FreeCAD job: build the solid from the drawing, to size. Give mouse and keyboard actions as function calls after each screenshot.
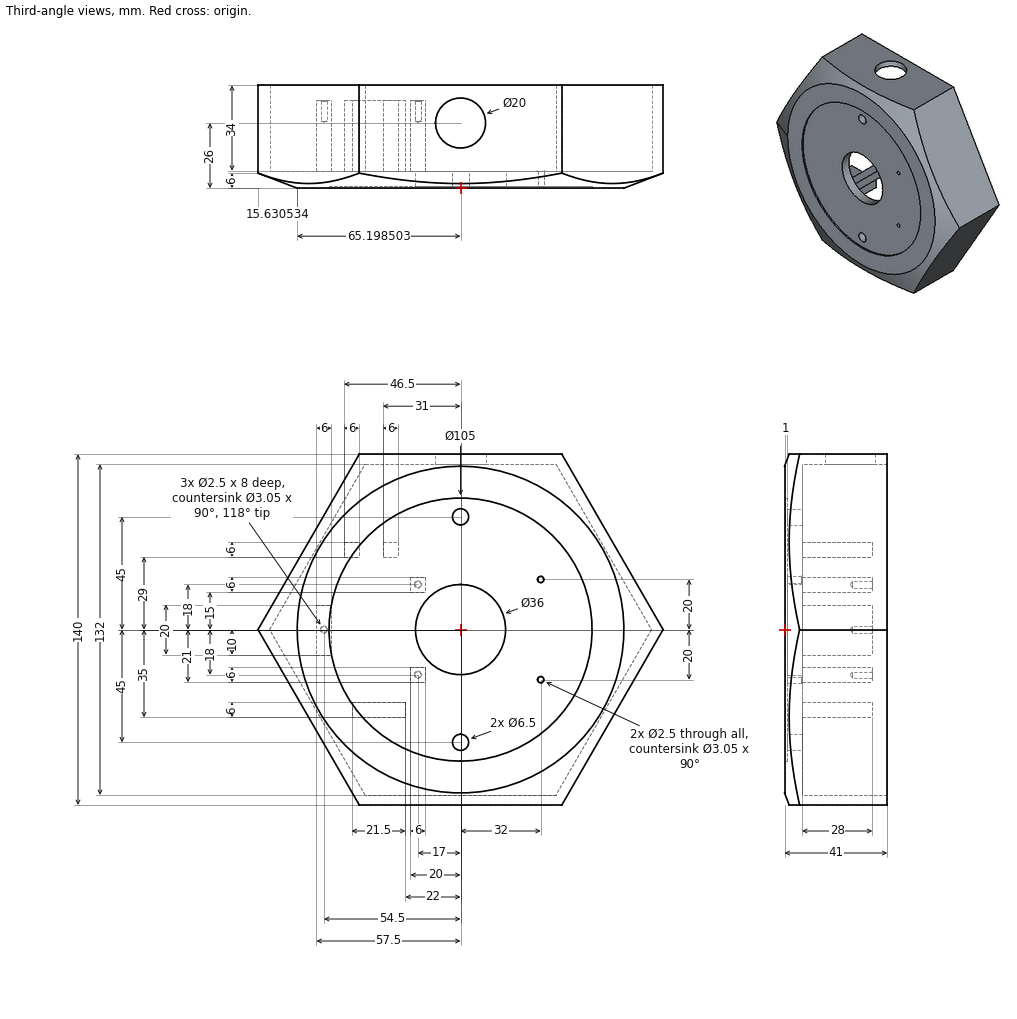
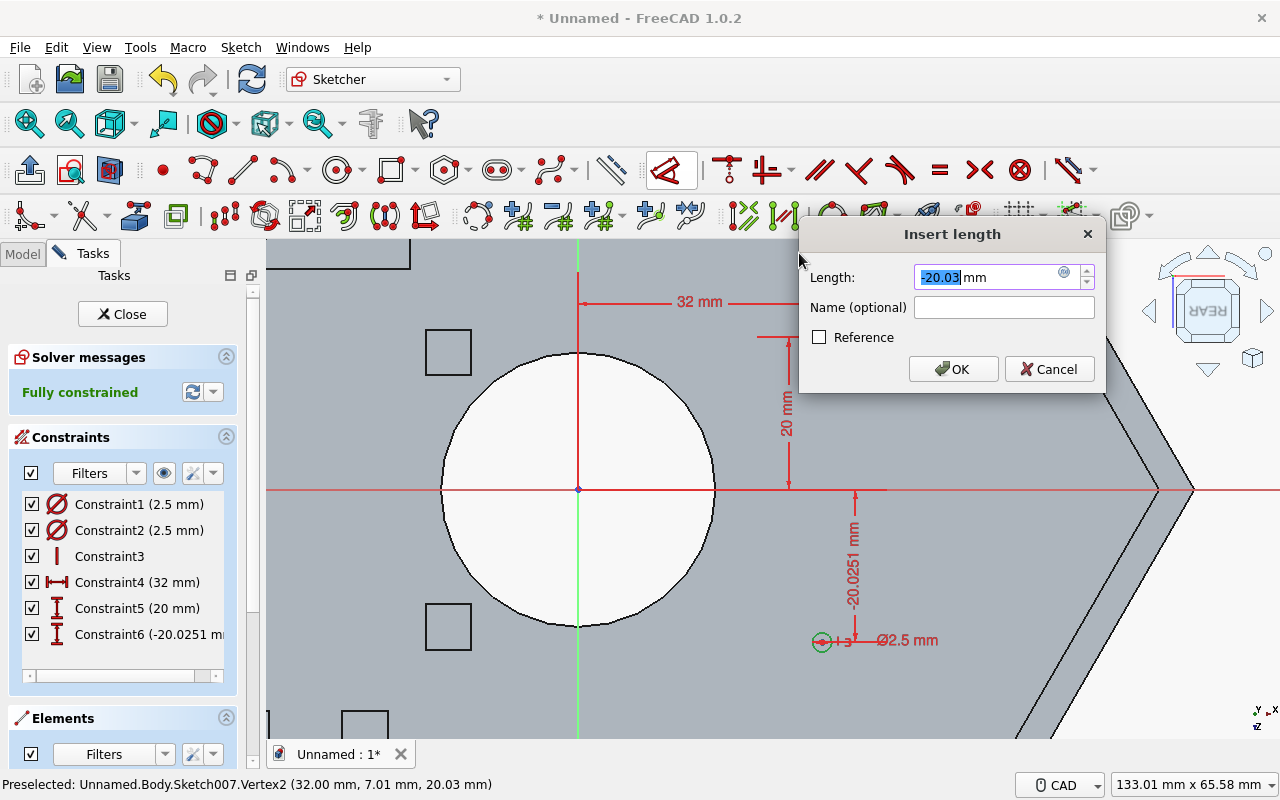
text(-20)
key(Return)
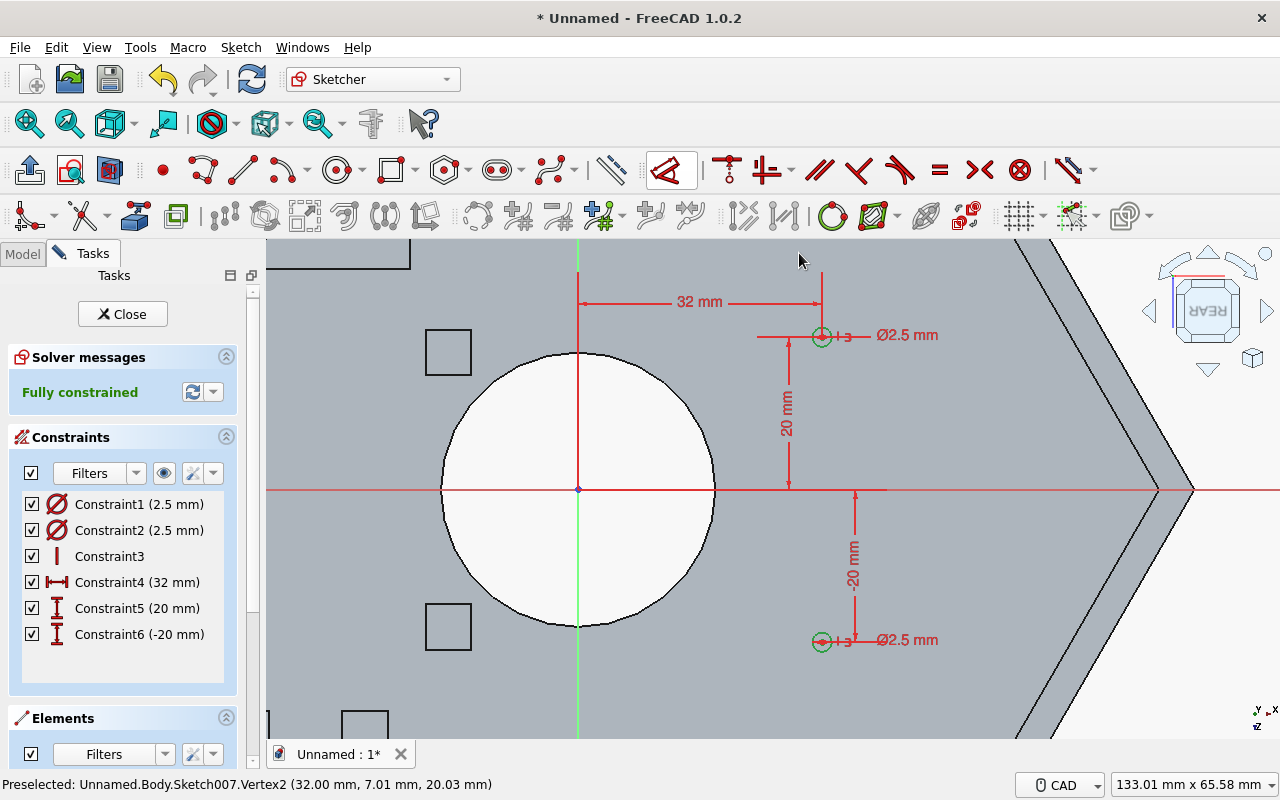
click(123, 314)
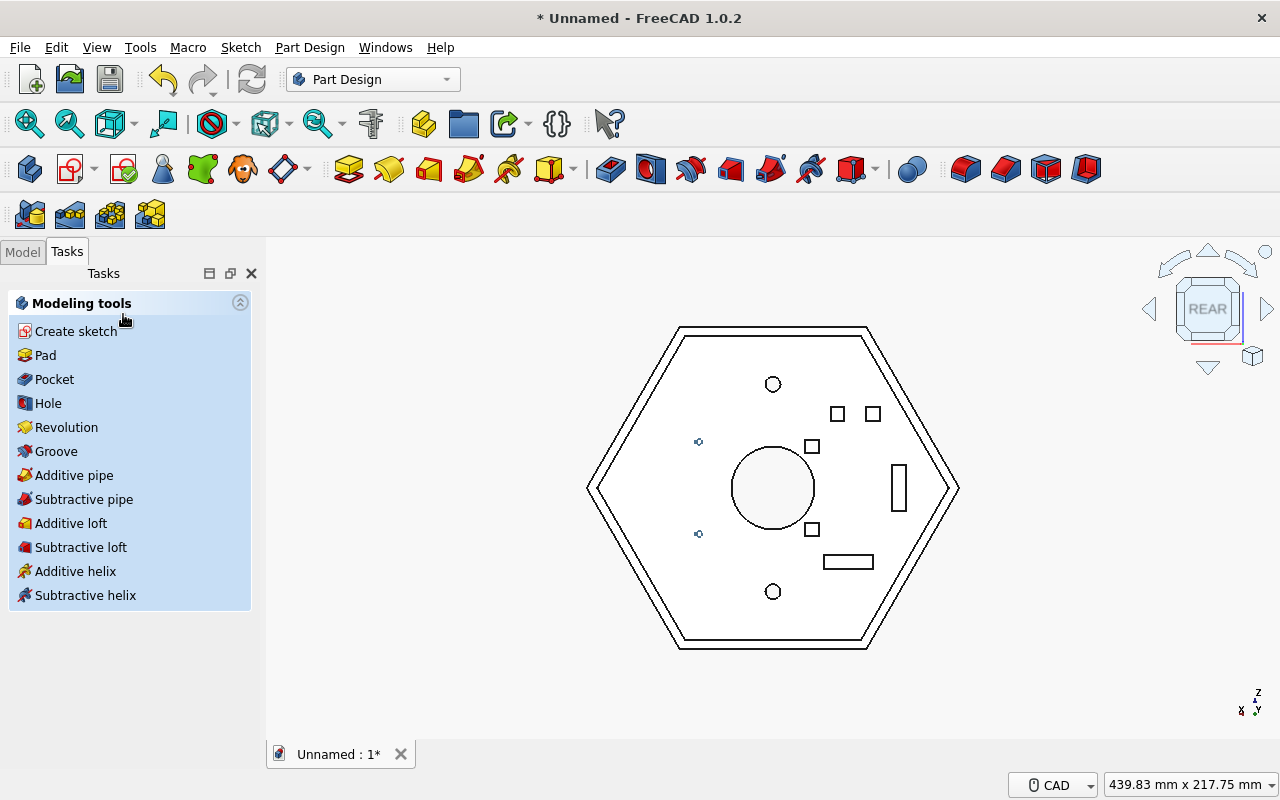
click(652, 170)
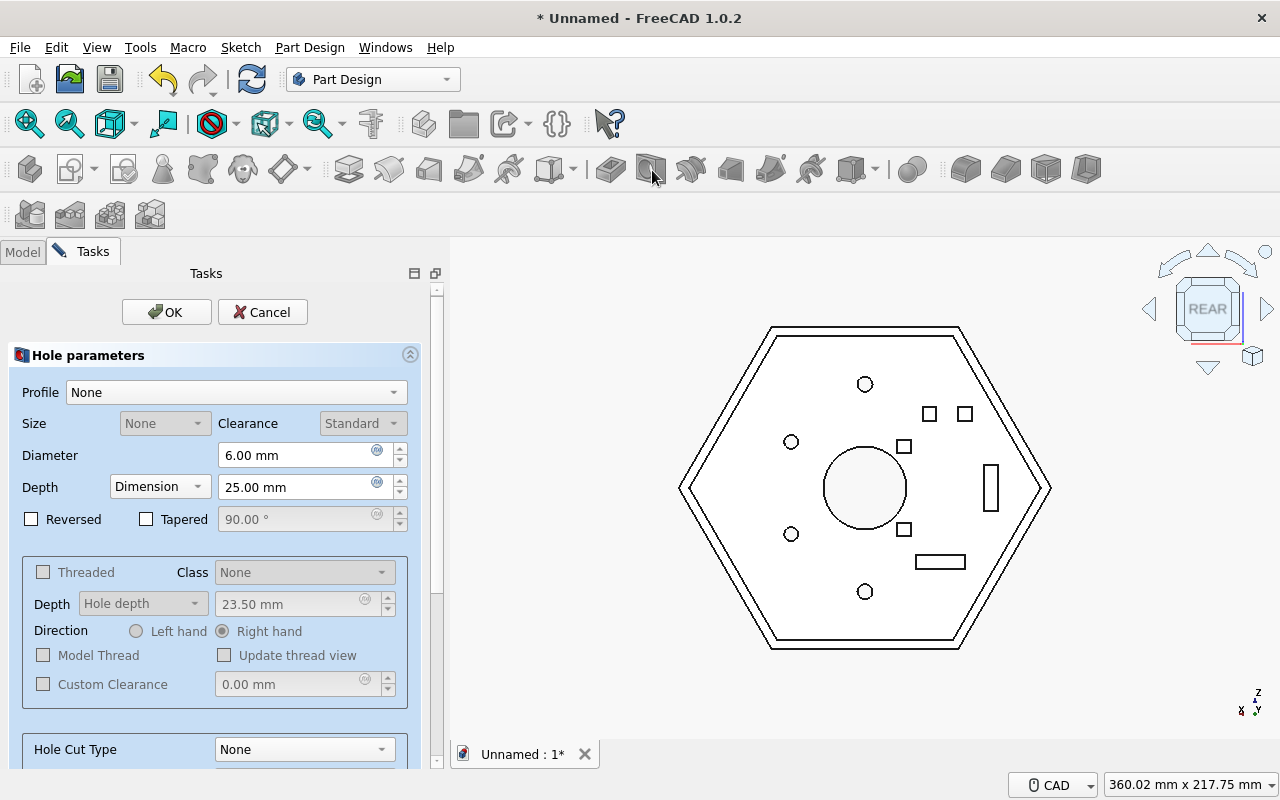
triple_click(305, 455)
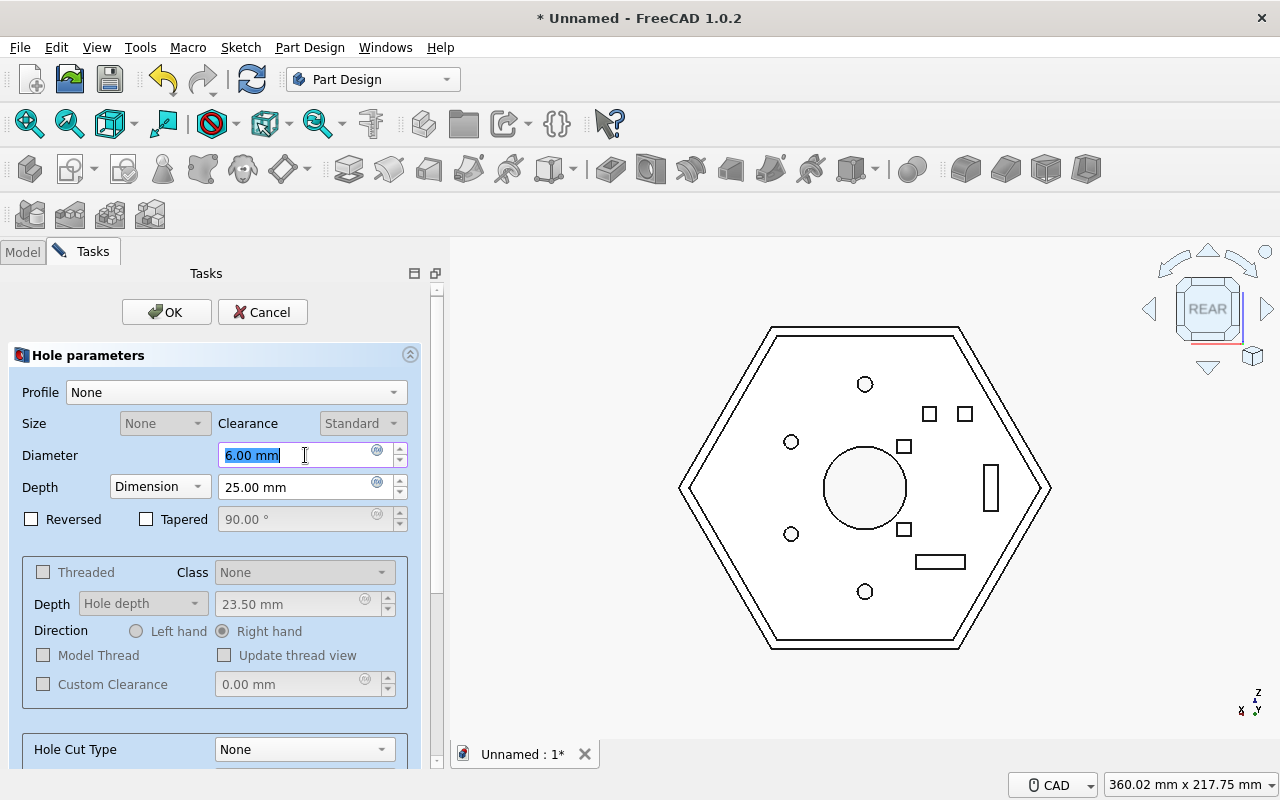
text(2.5)
key(Tab)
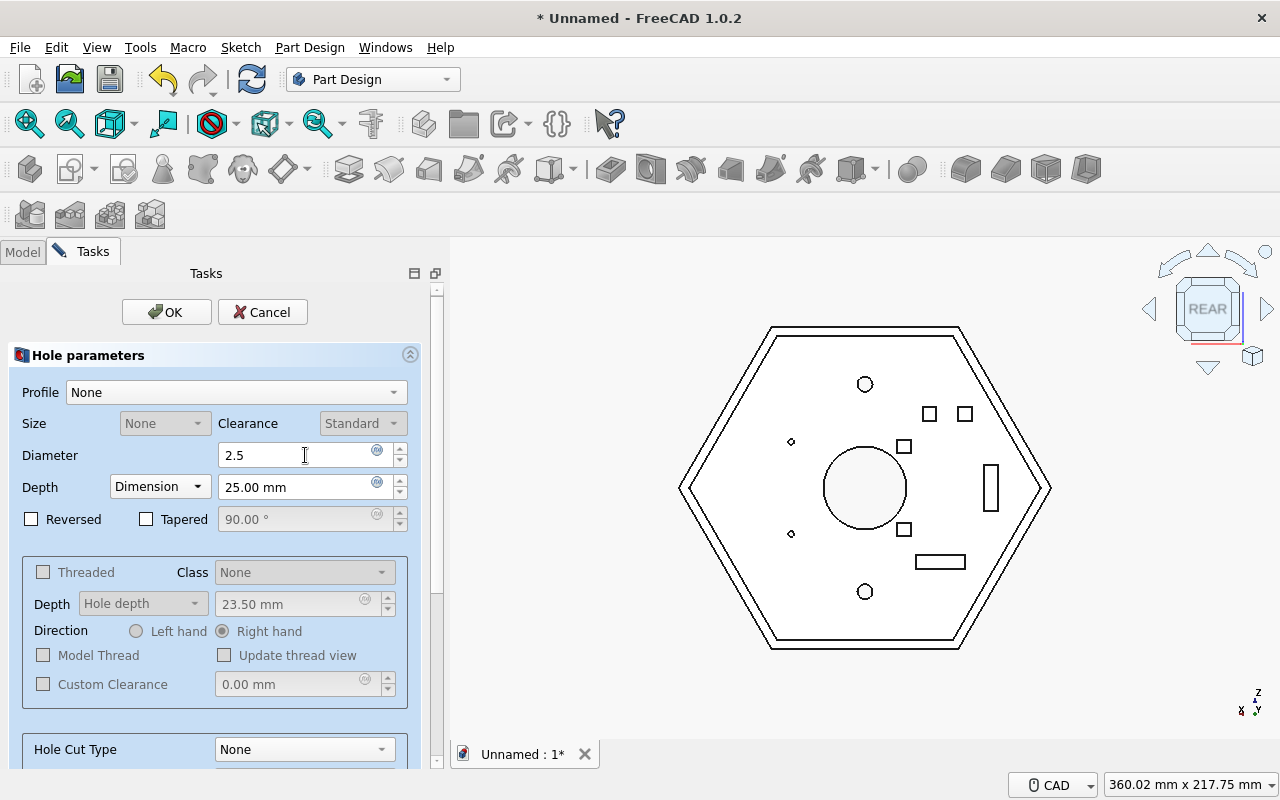
click(161, 486)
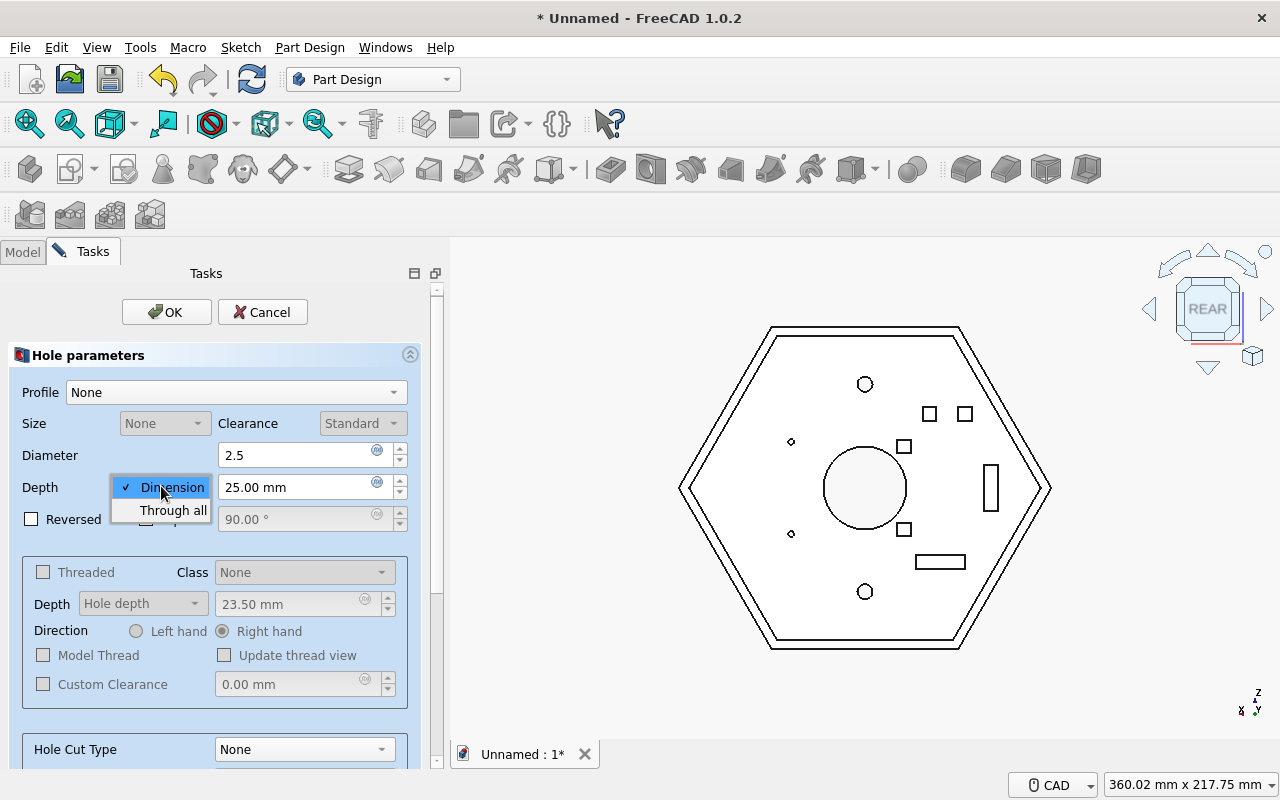
click(160, 510)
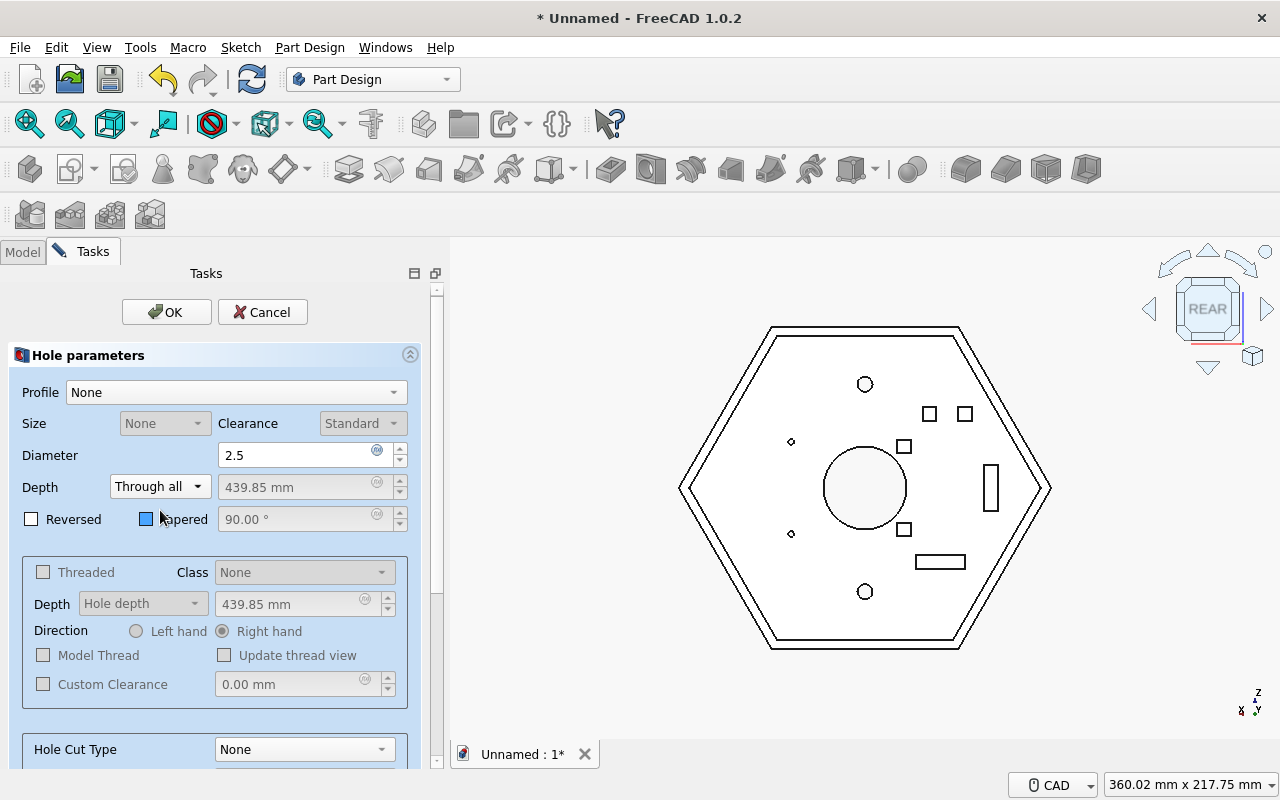
click(306, 750)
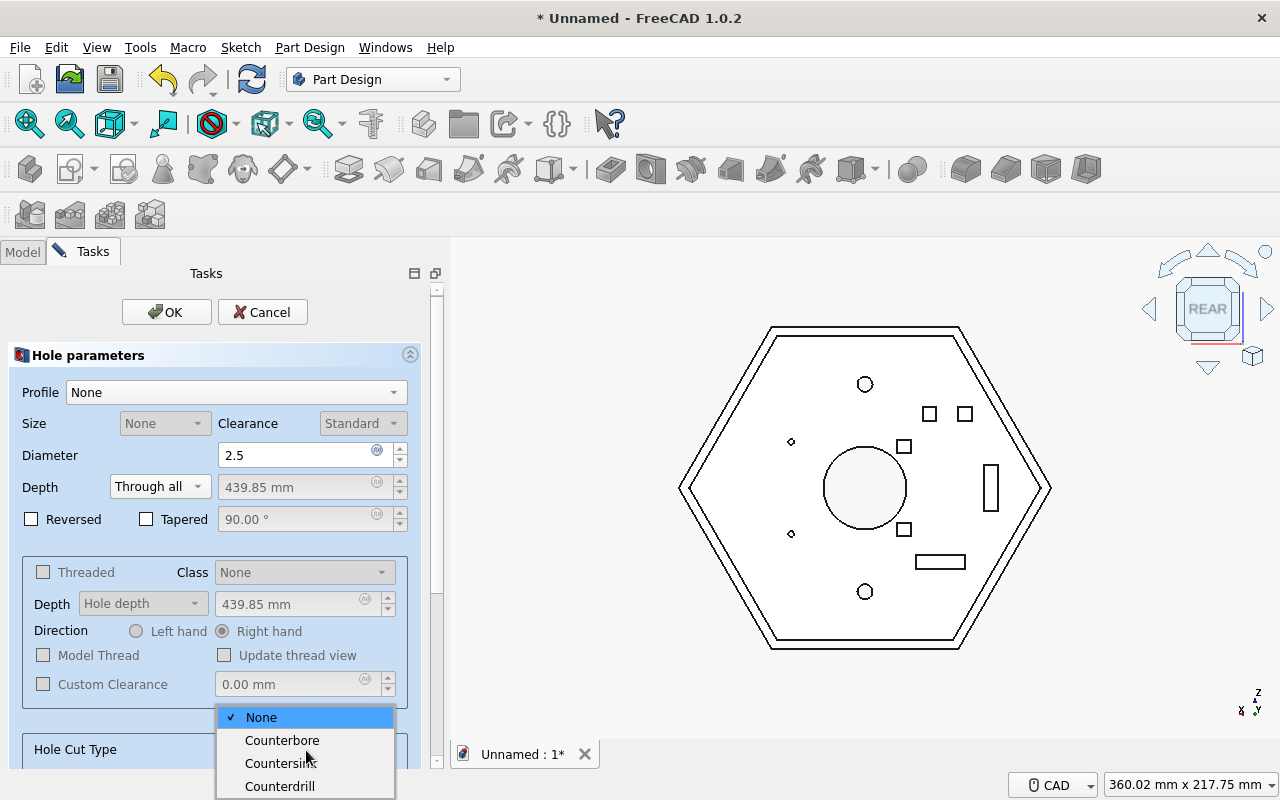
click(304, 764)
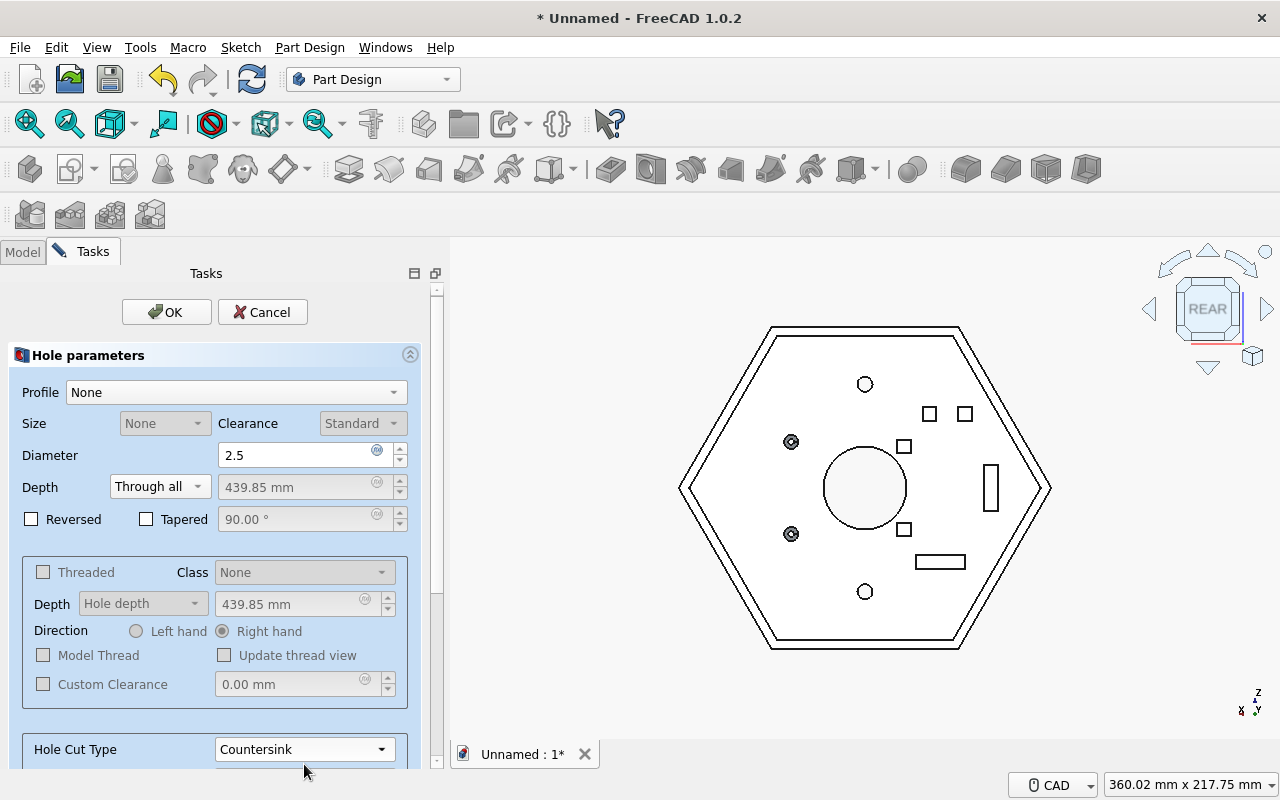
scroll(437, 526, down, 2)